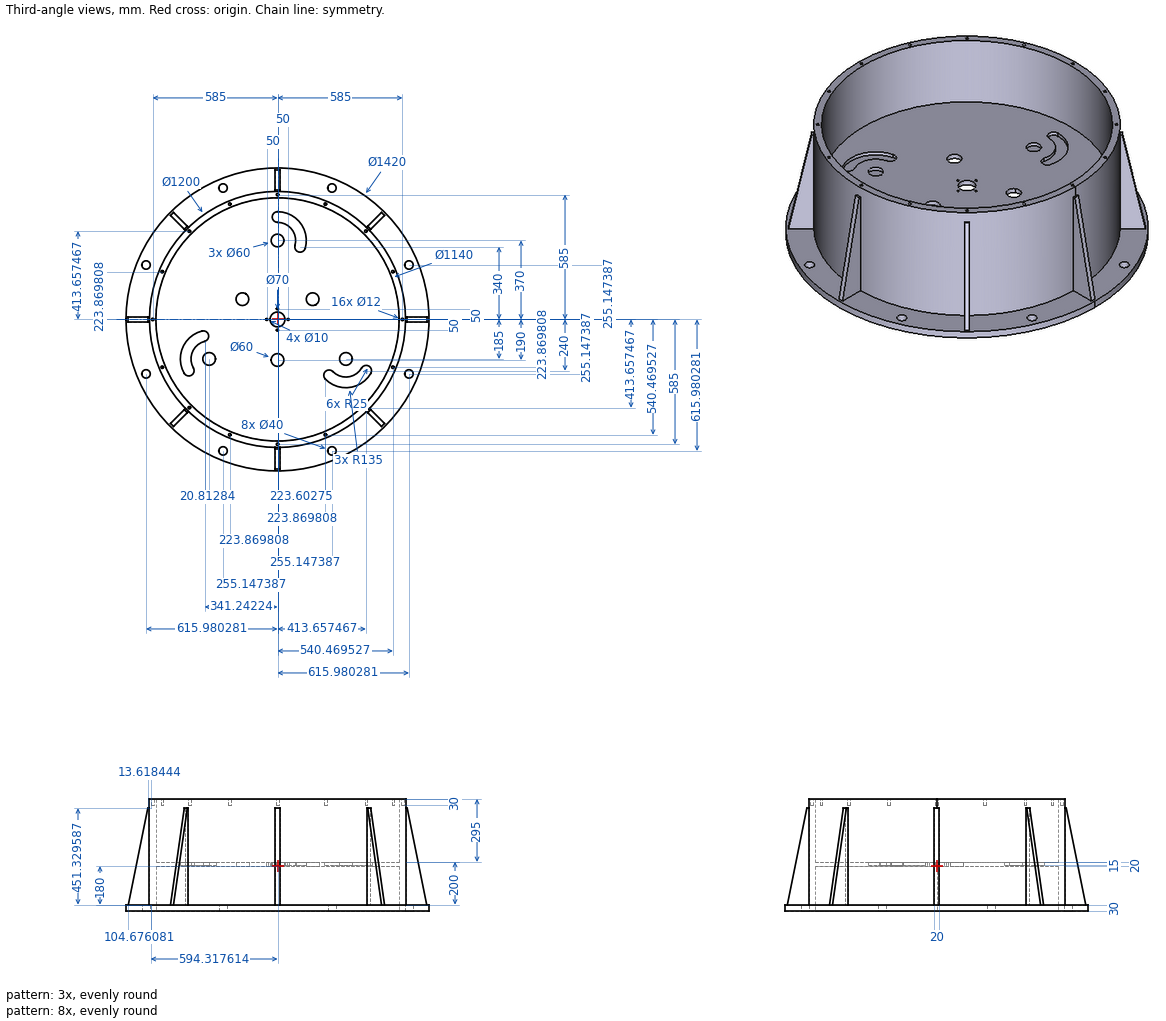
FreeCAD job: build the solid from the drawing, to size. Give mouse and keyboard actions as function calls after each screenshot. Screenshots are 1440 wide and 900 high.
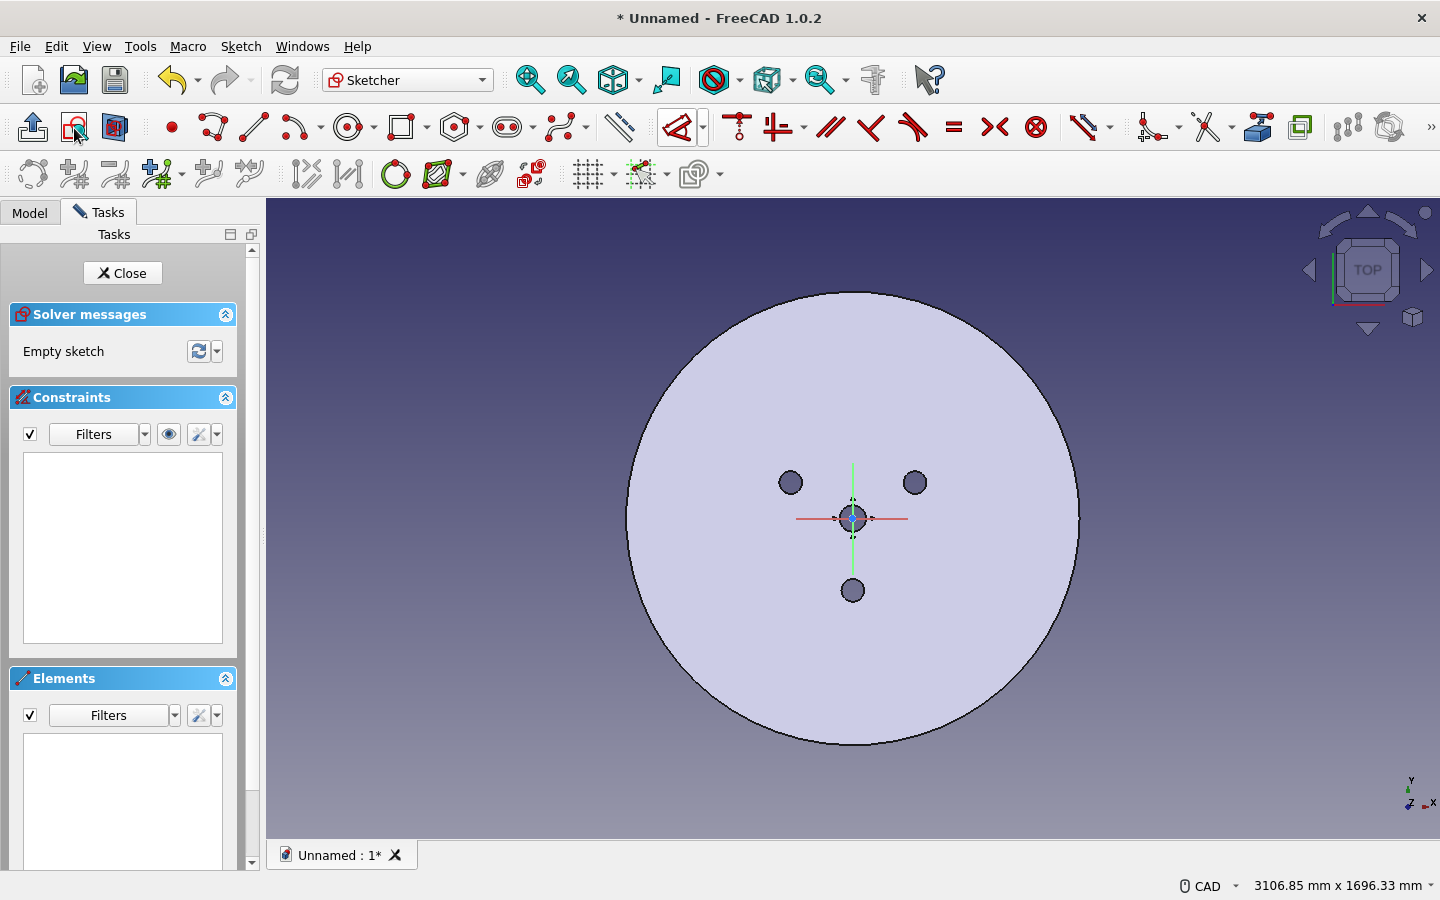
key(g)
key(3)
key(a)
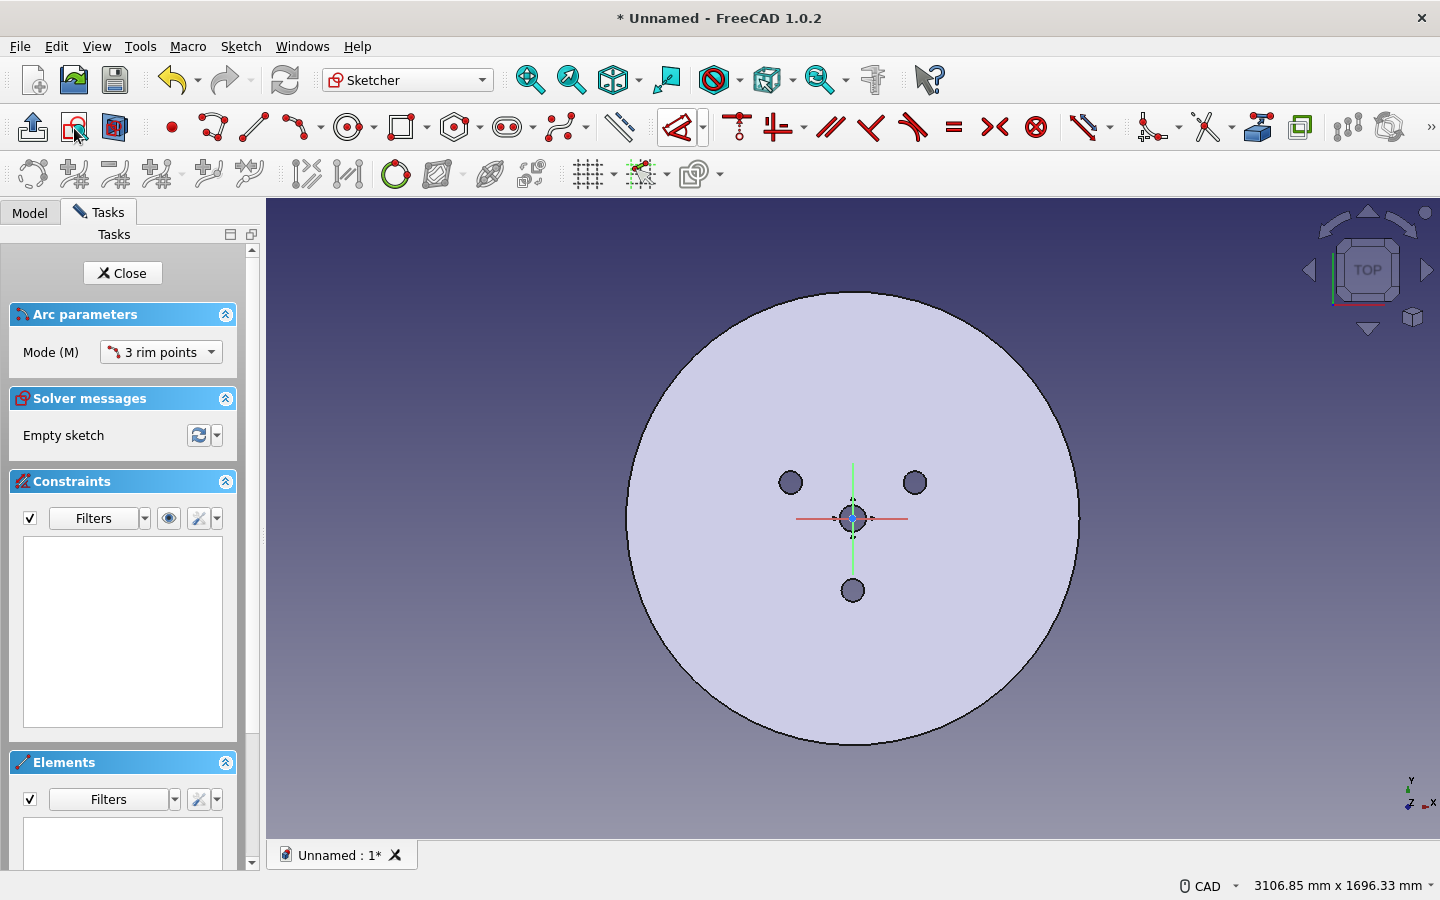
click(951, 611)
click(937, 624)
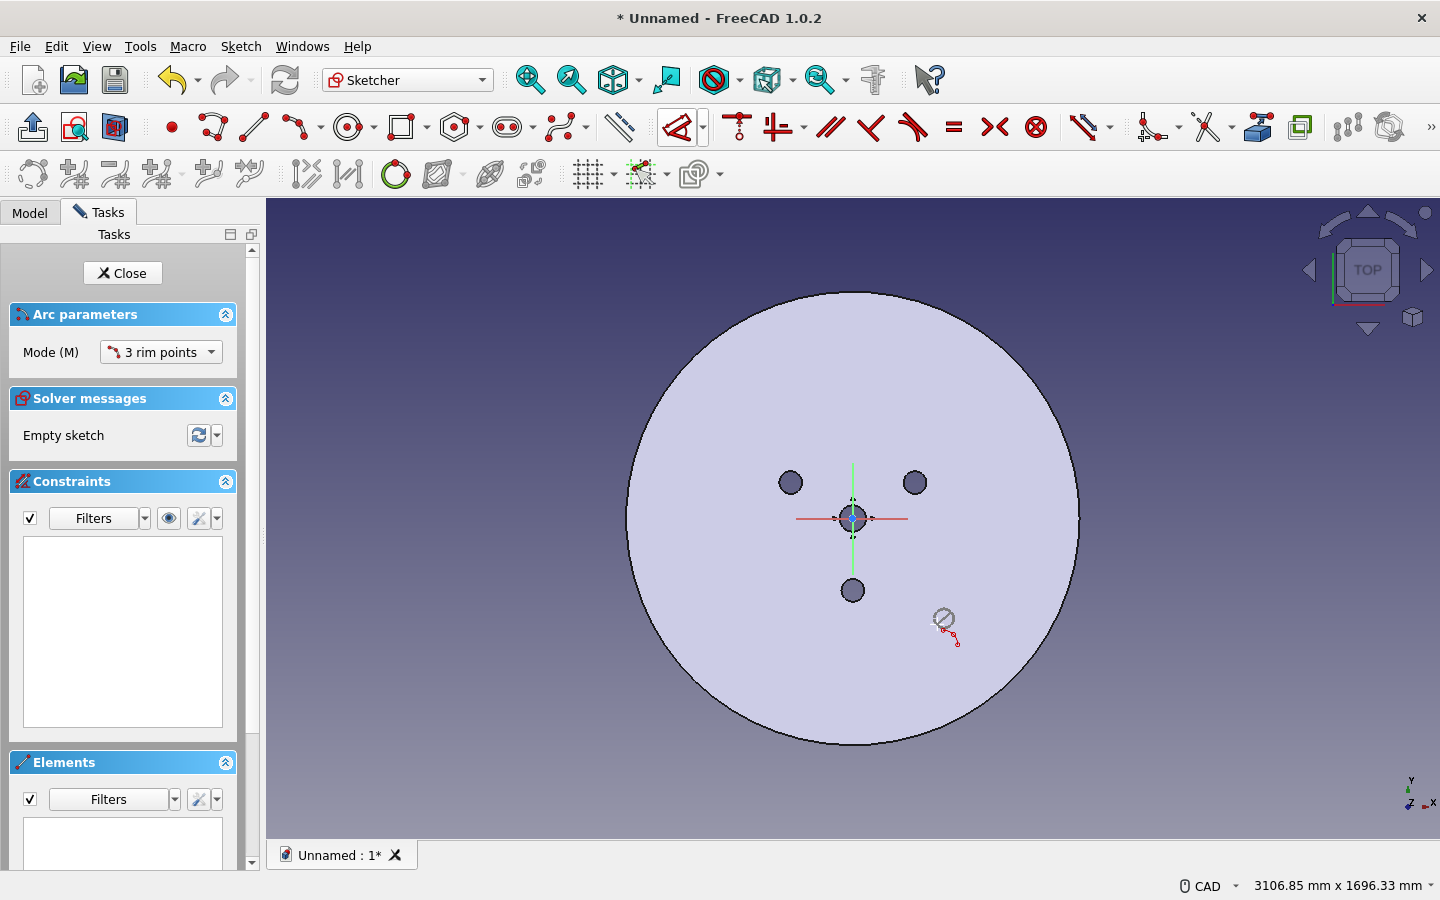
scroll(938, 611, up, 3)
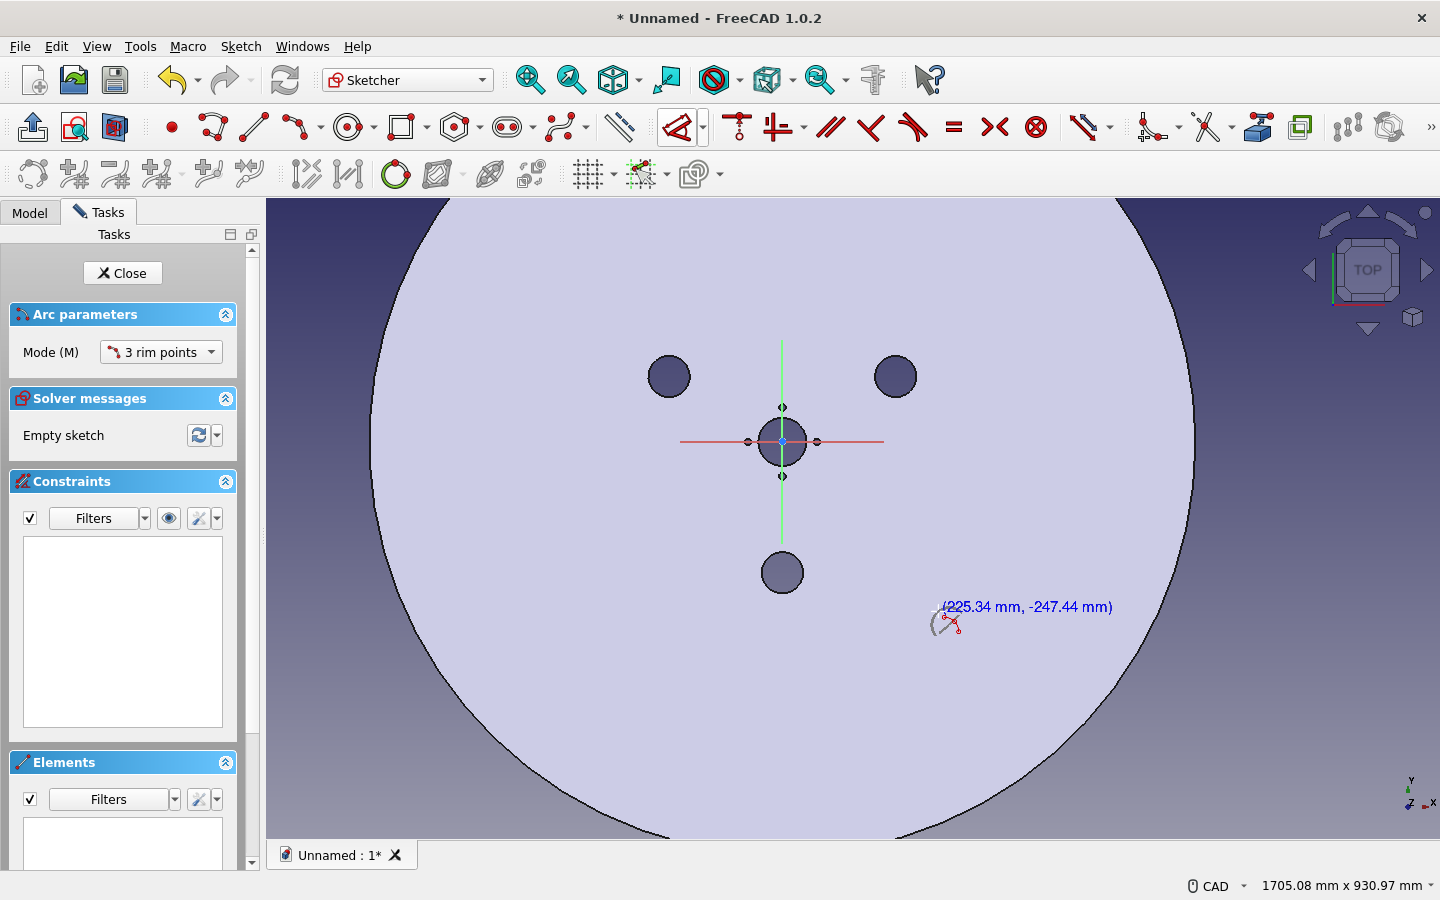
click(937, 610)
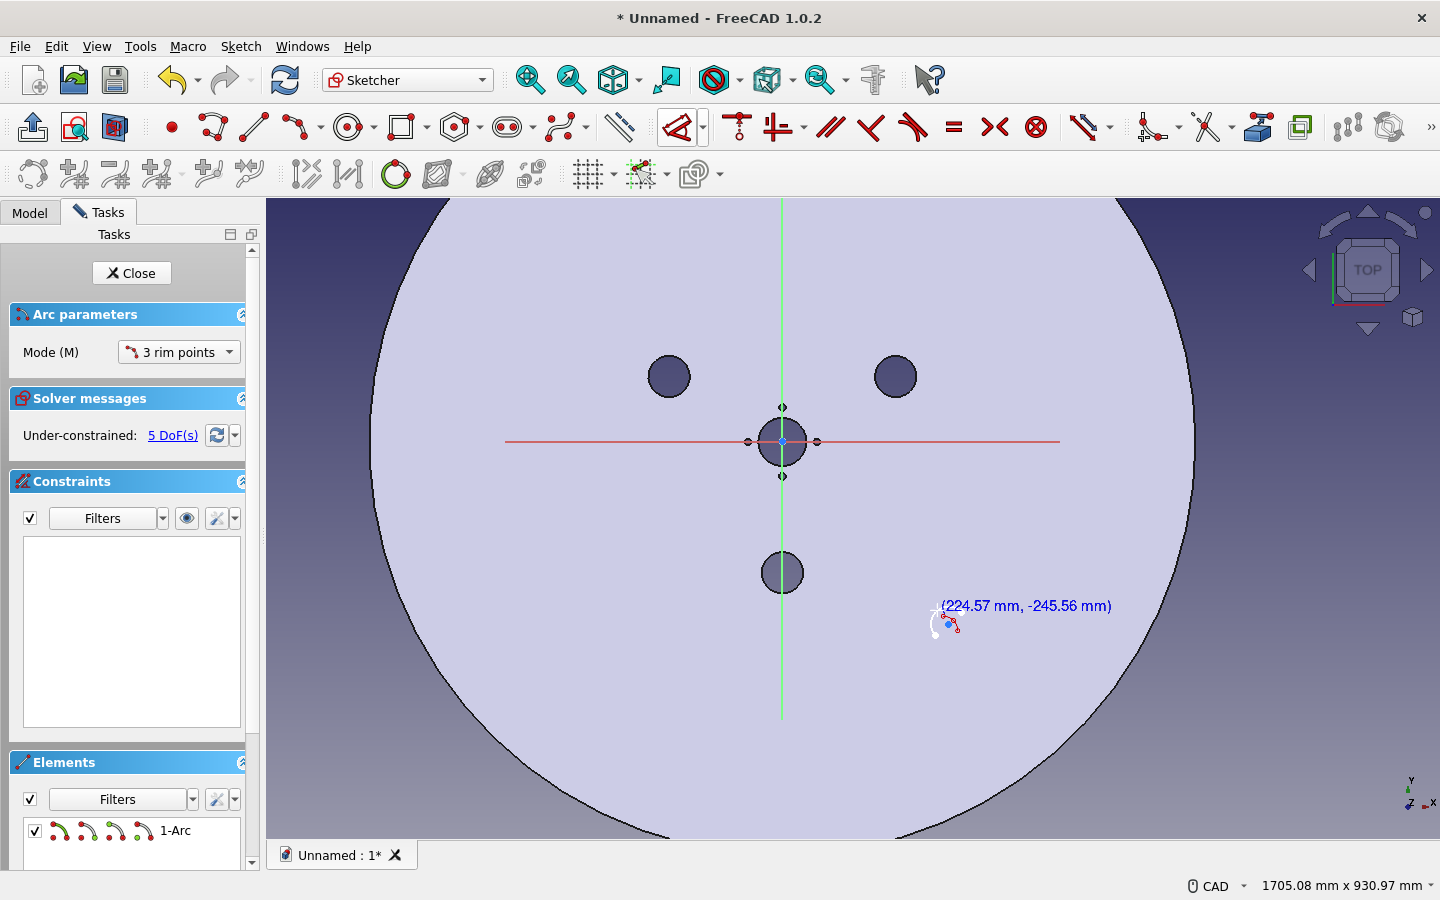
click(936, 636)
click(1083, 616)
click(1014, 662)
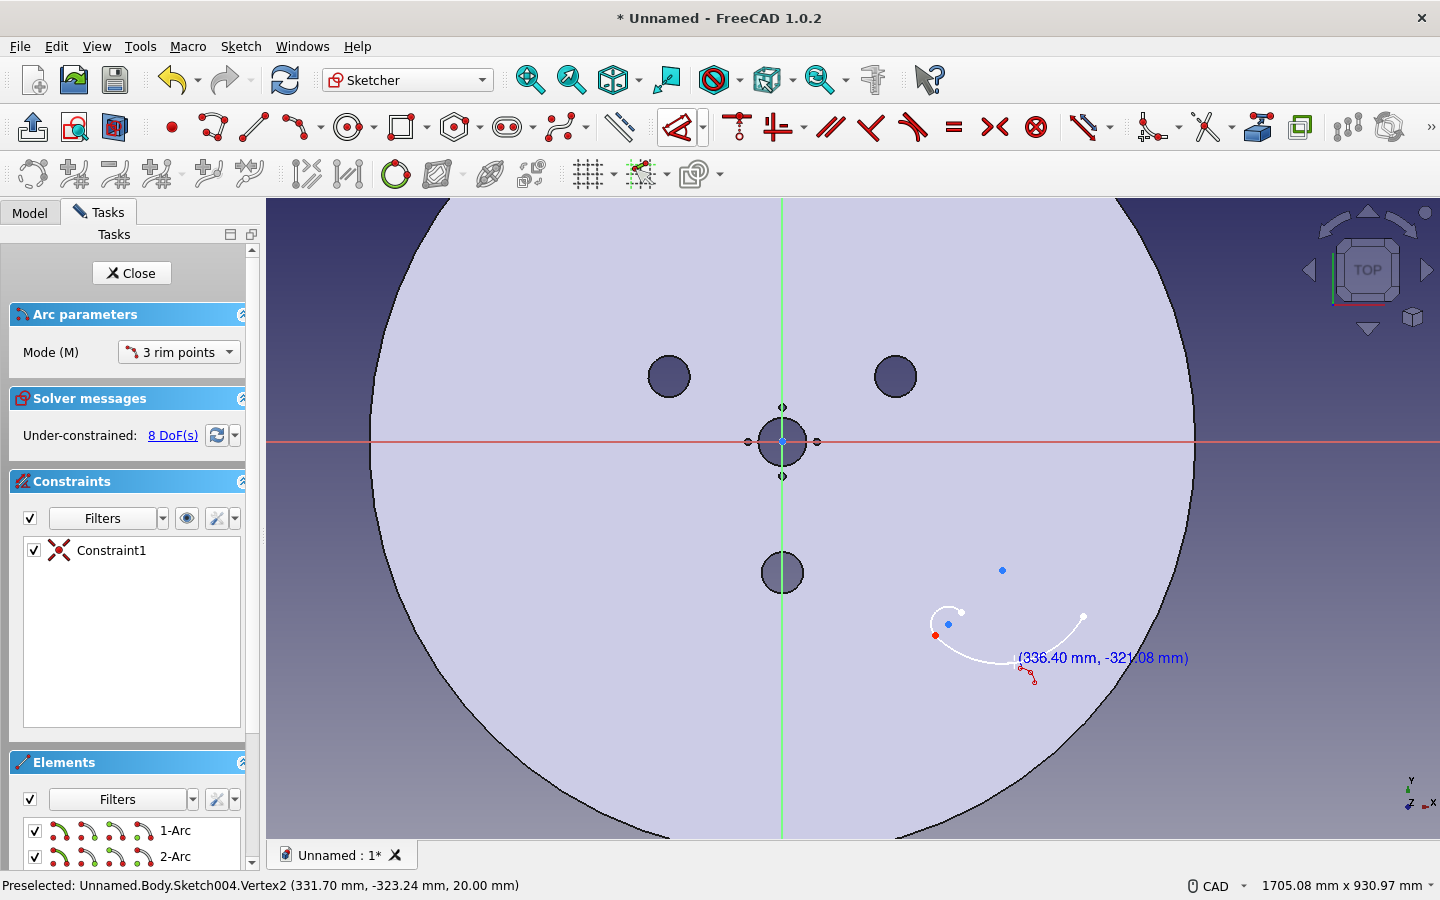
click(1083, 617)
click(1054, 599)
click(1077, 592)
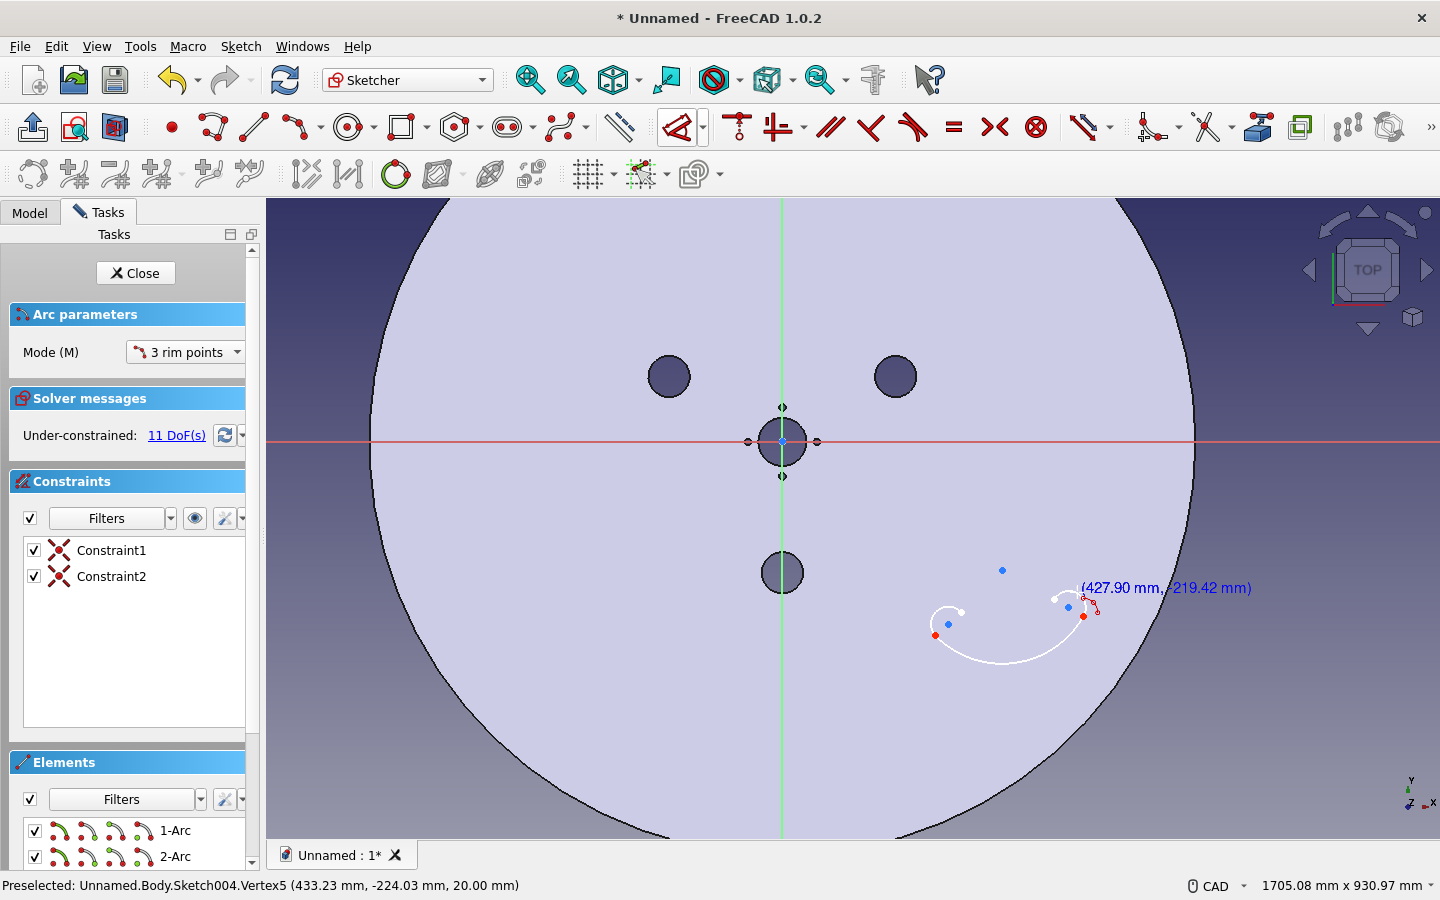
click(1054, 600)
click(961, 612)
click(1010, 627)